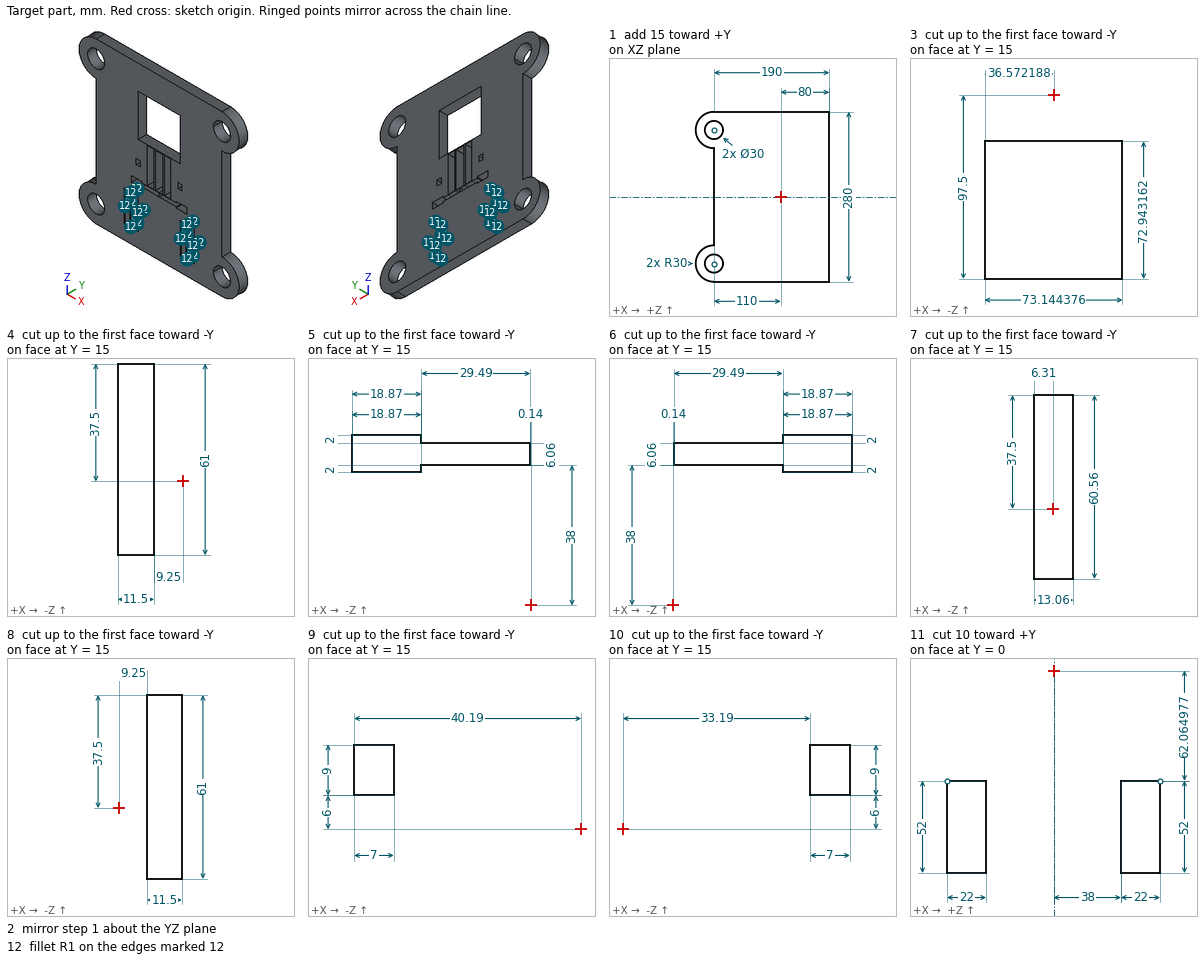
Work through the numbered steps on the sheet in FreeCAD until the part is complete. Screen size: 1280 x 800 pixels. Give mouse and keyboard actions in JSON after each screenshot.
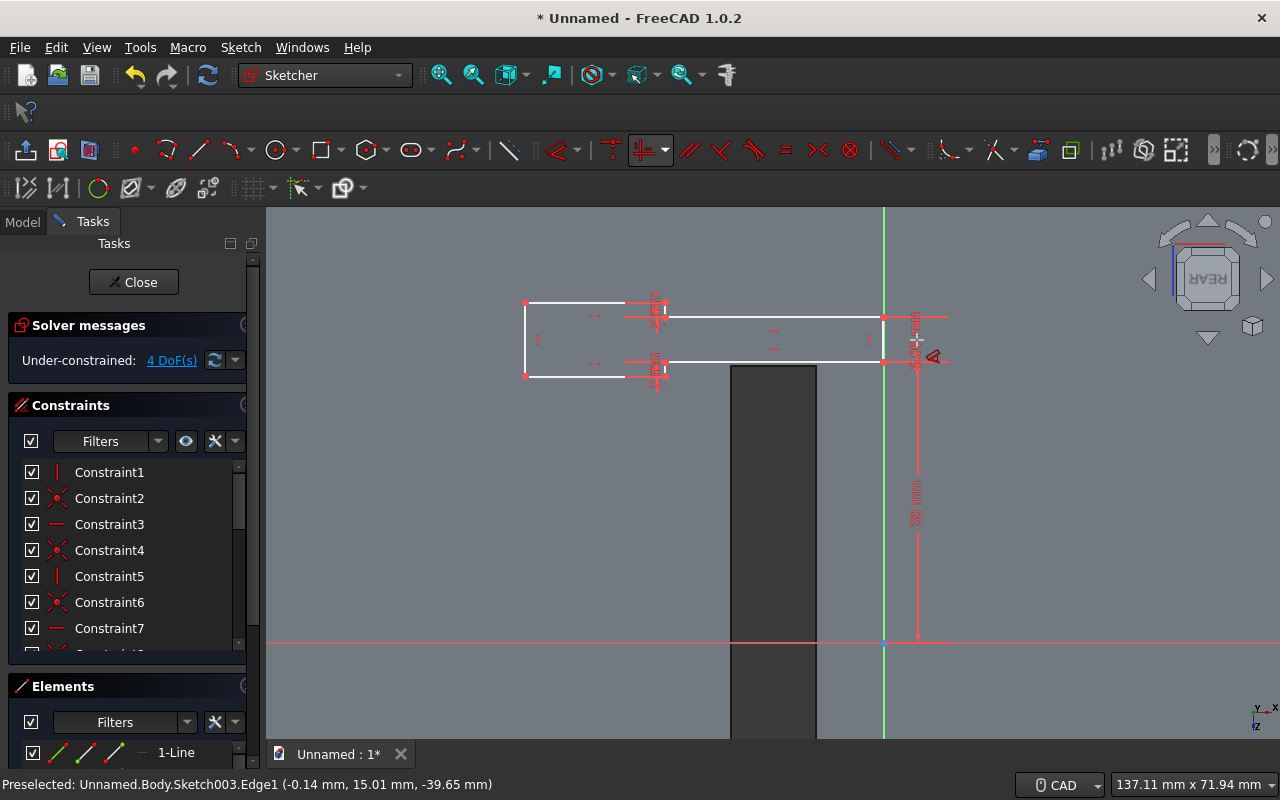
{"action": "left_click", "coordinate": [818, 317]}
{"action": "left_click", "coordinate": [774, 283]}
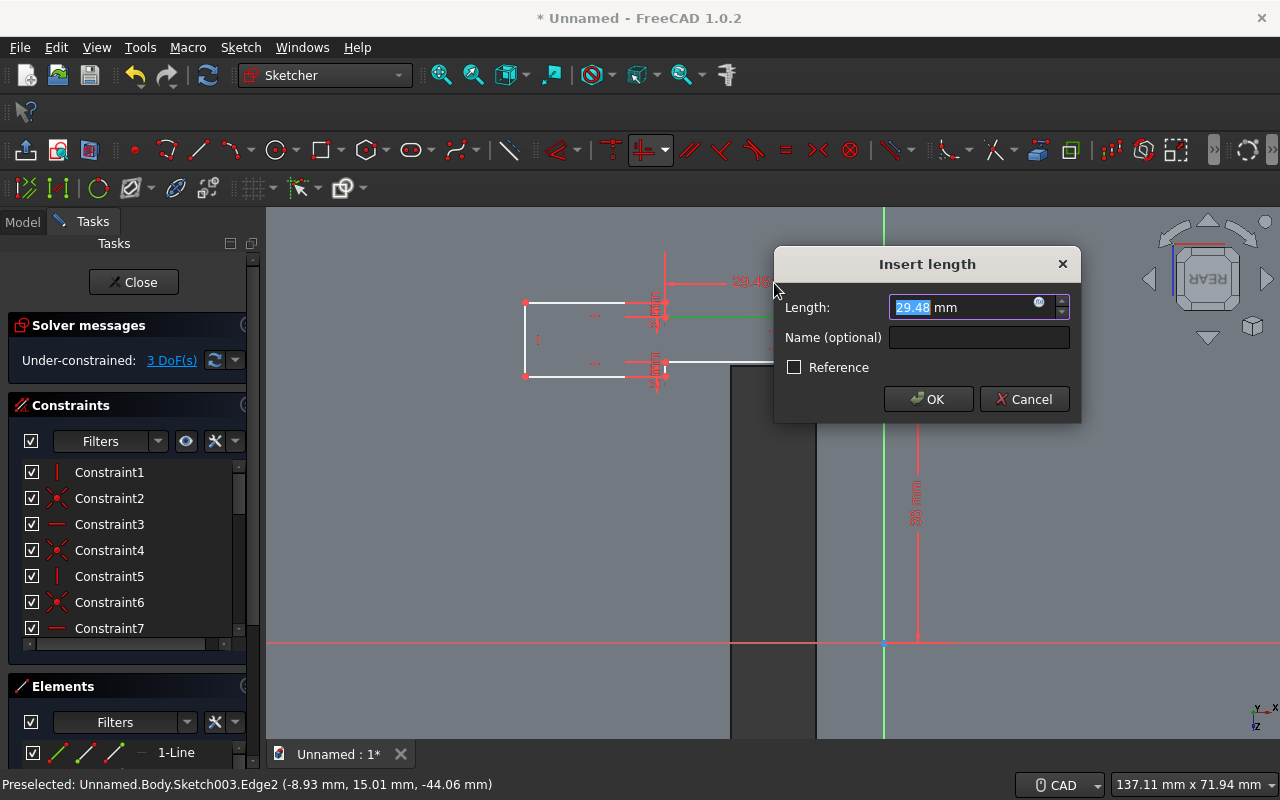
{"action": "type", "text": "29.49"}
{"action": "key", "text": "Return"}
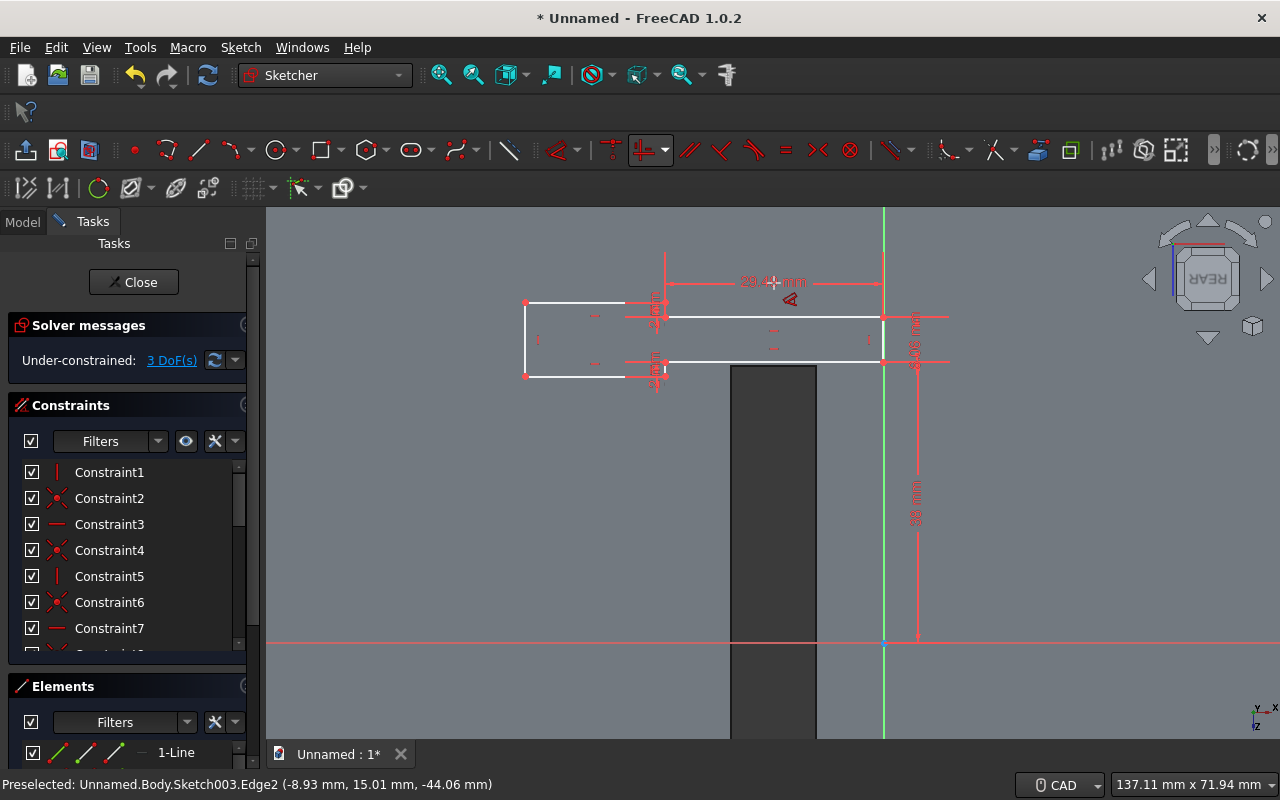
{"action": "left_click", "coordinate": [623, 303]}
{"action": "left_click", "coordinate": [595, 269]}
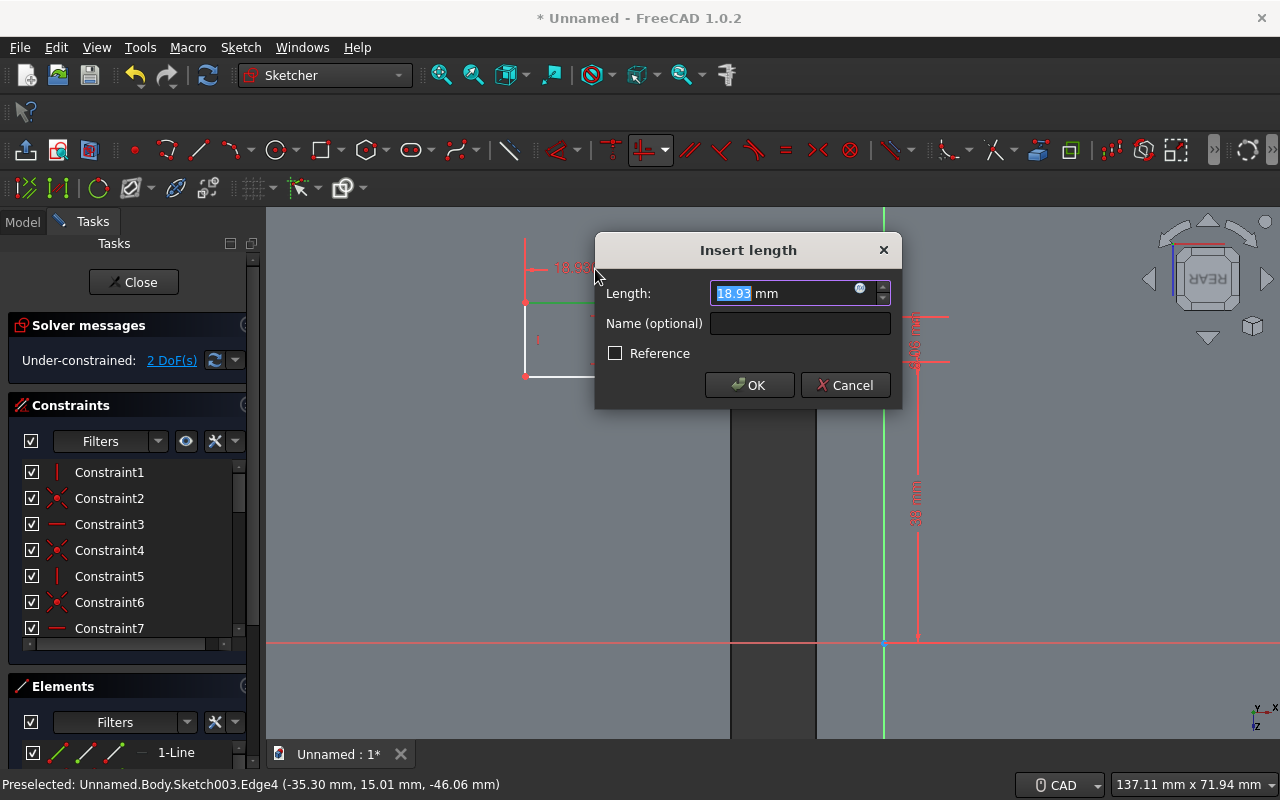
{"action": "type", "text": "18.87"}
{"action": "key", "text": "Return"}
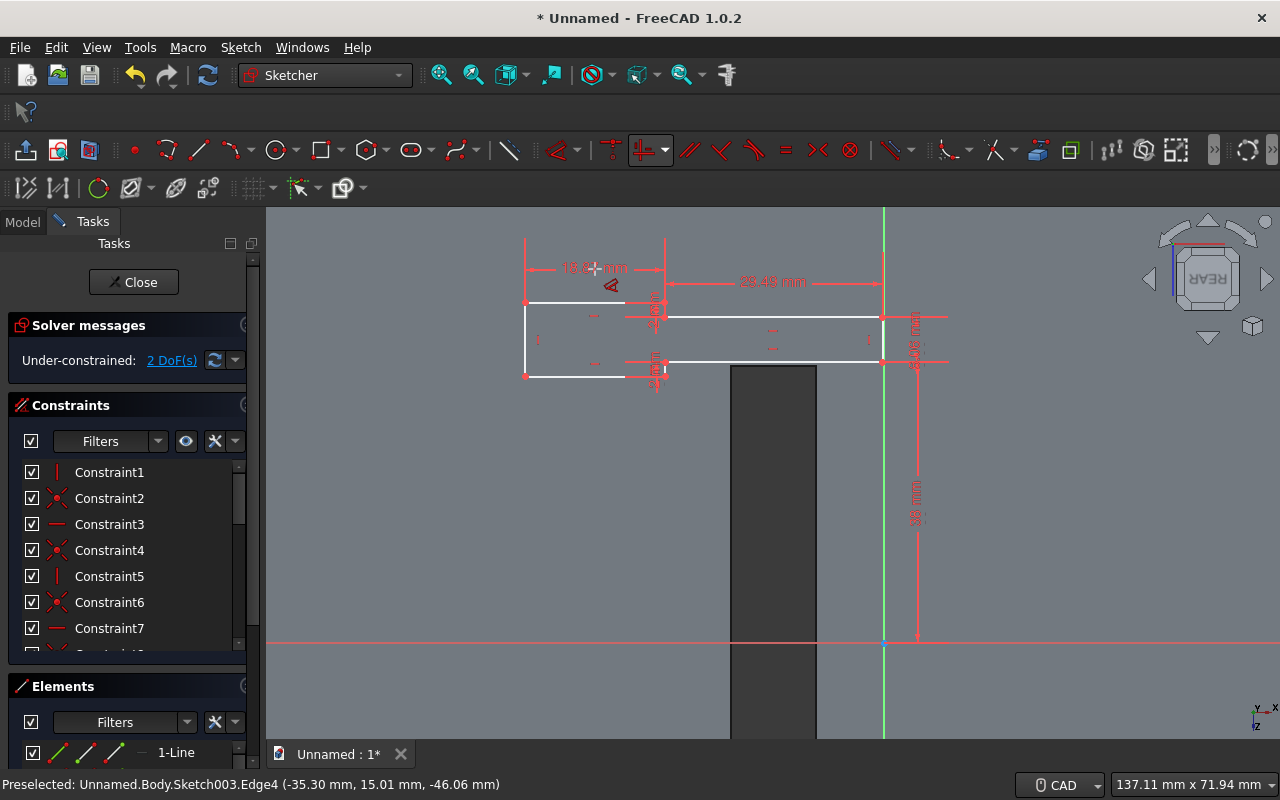
{"action": "left_click", "coordinate": [567, 377]}
{"action": "left_click", "coordinate": [595, 343]}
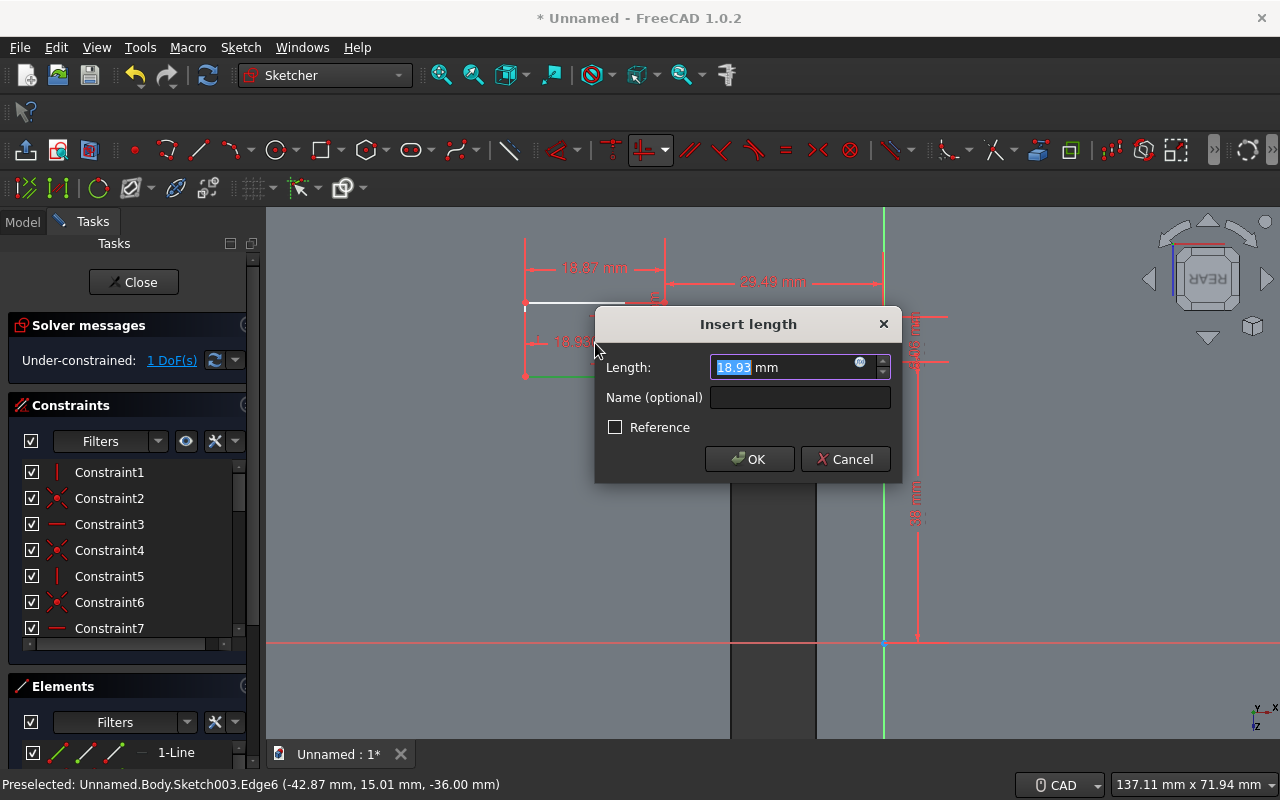
{"action": "type", "text": "18.87"}
{"action": "key", "text": "Return"}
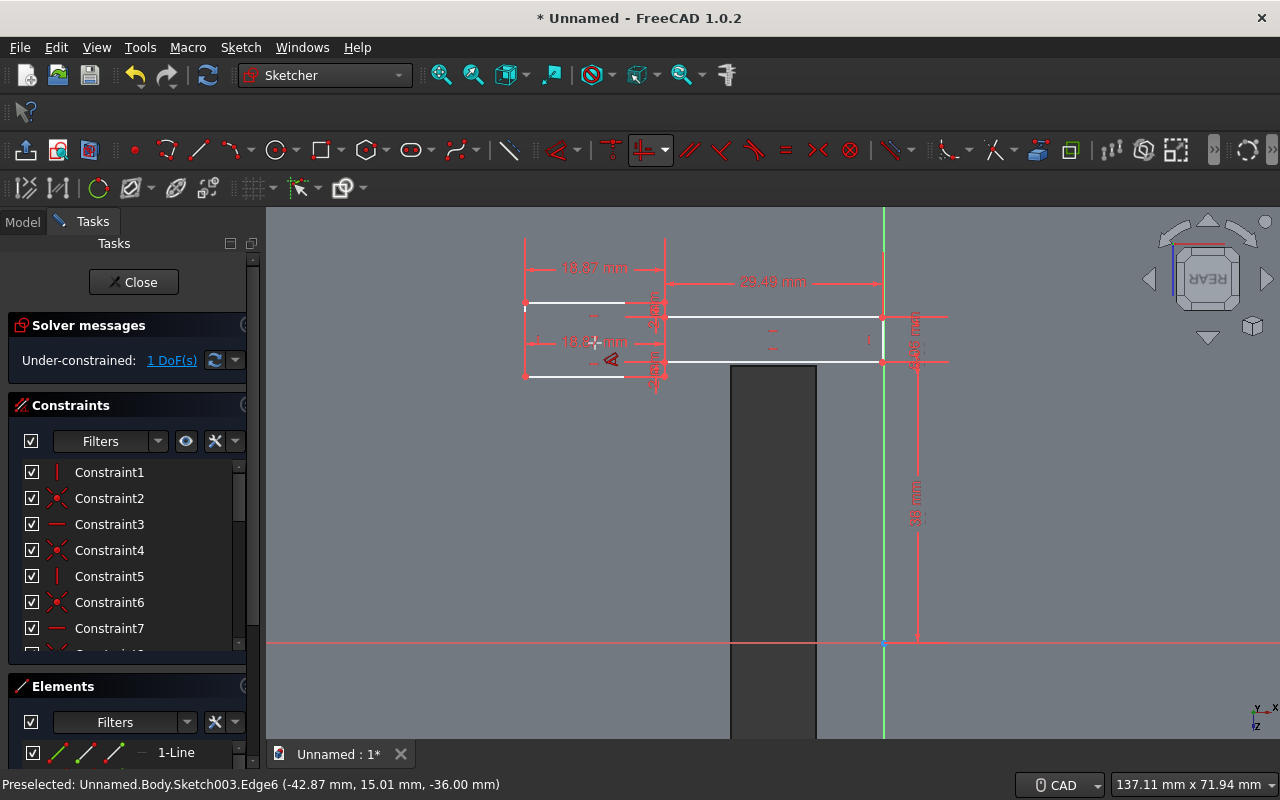
{"action": "scroll", "coordinate": [883, 362], "scroll_direction": "up", "scroll_amount": 19}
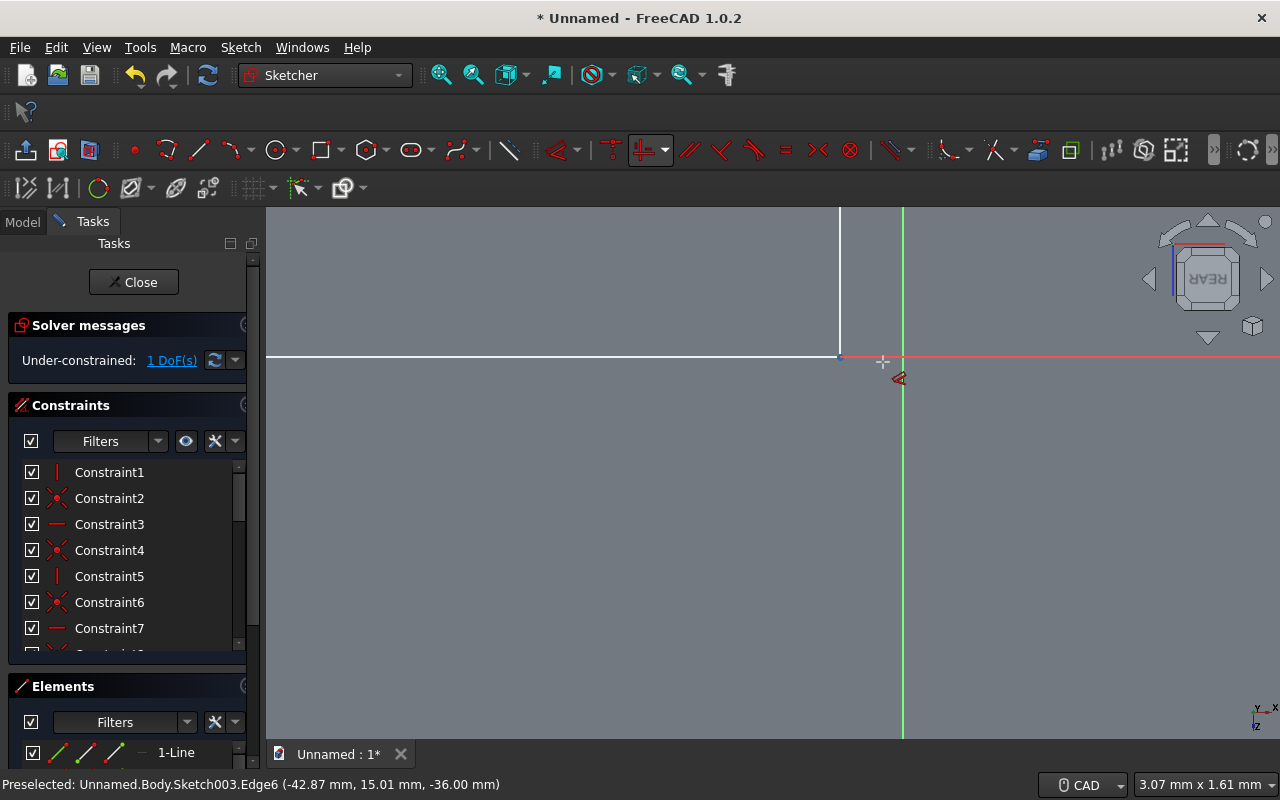
{"action": "left_click", "coordinate": [840, 357]}
{"action": "left_click", "coordinate": [872, 323]}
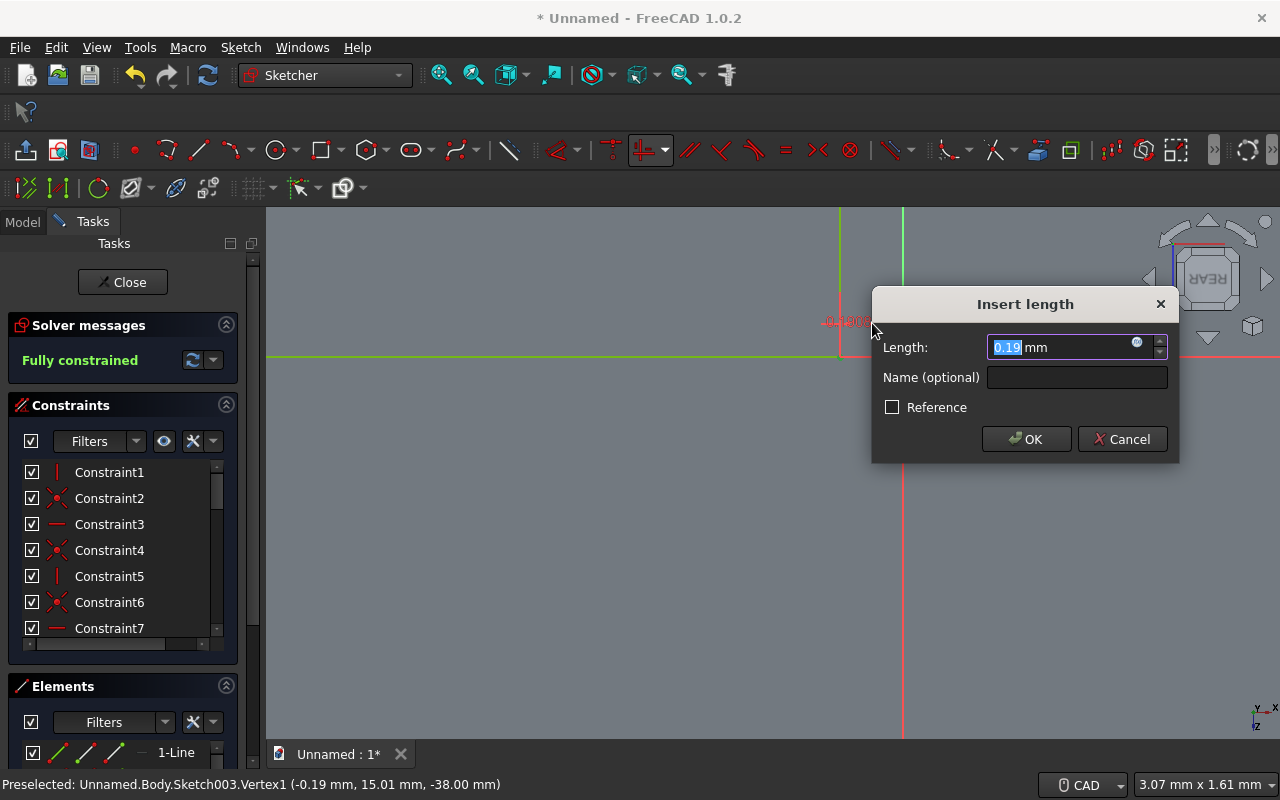
{"action": "type", "text": "0.14"}
{"action": "key", "text": "Return"}
{"action": "key", "text": "Escape"}